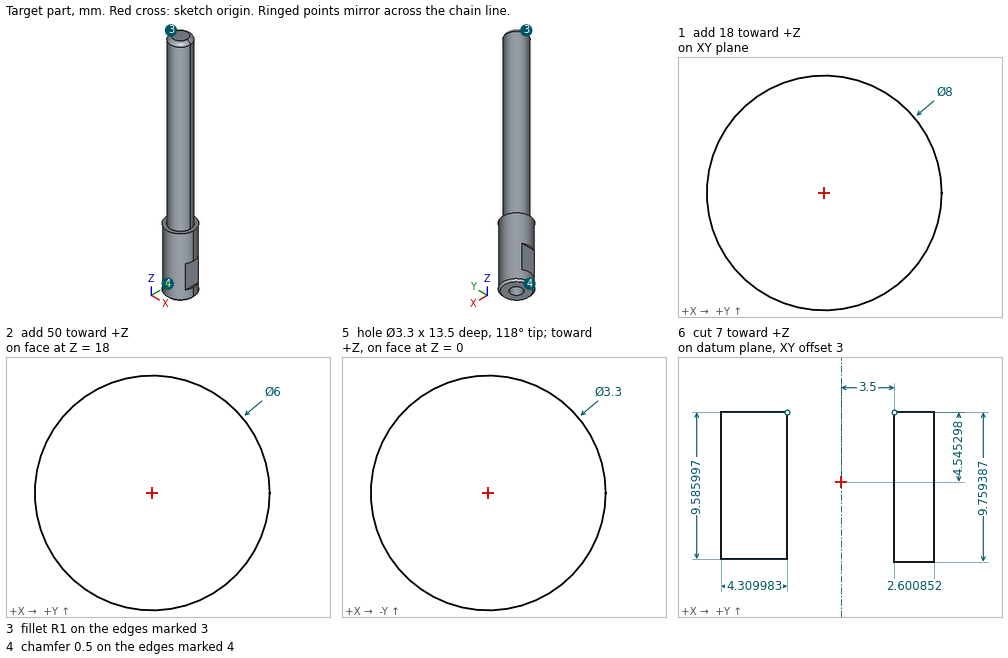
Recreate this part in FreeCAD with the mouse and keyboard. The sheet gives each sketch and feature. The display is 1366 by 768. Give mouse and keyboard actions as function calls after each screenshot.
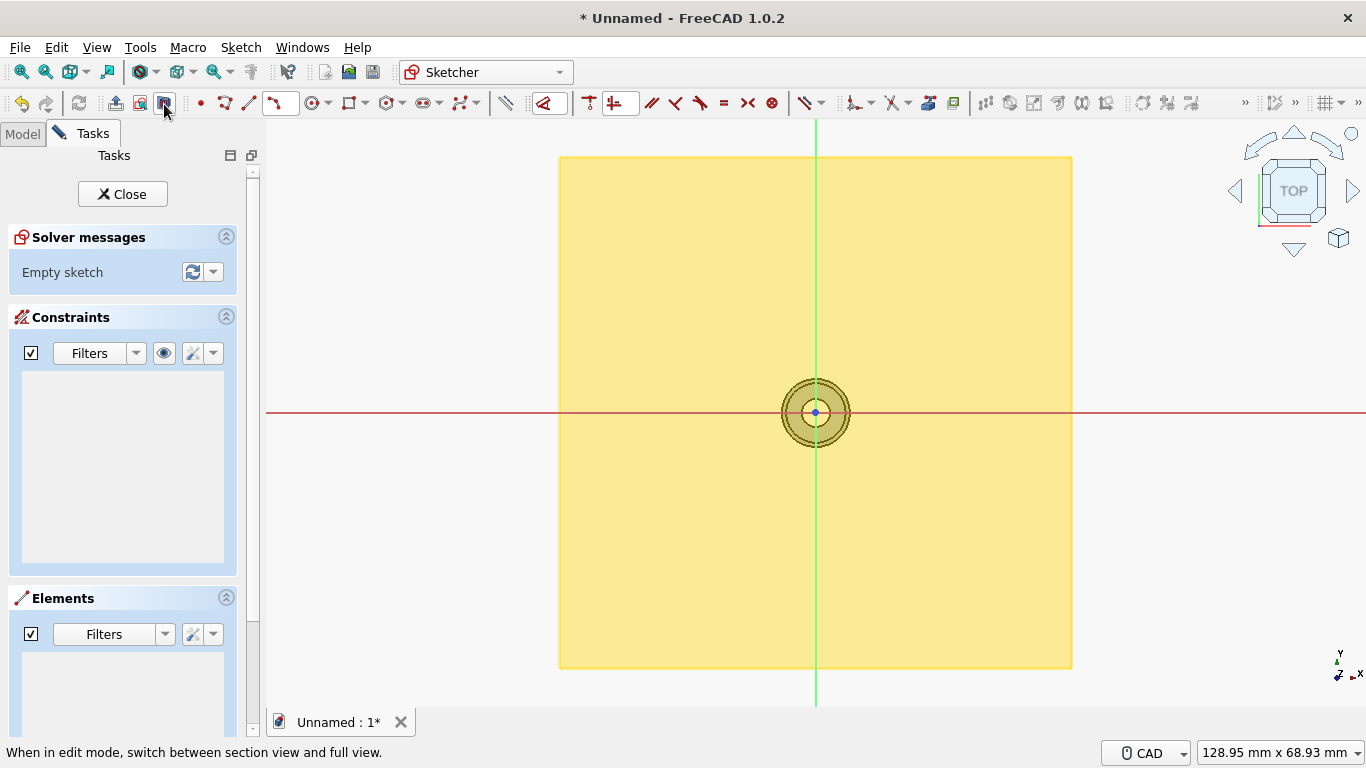
scroll(824, 417, up, 8)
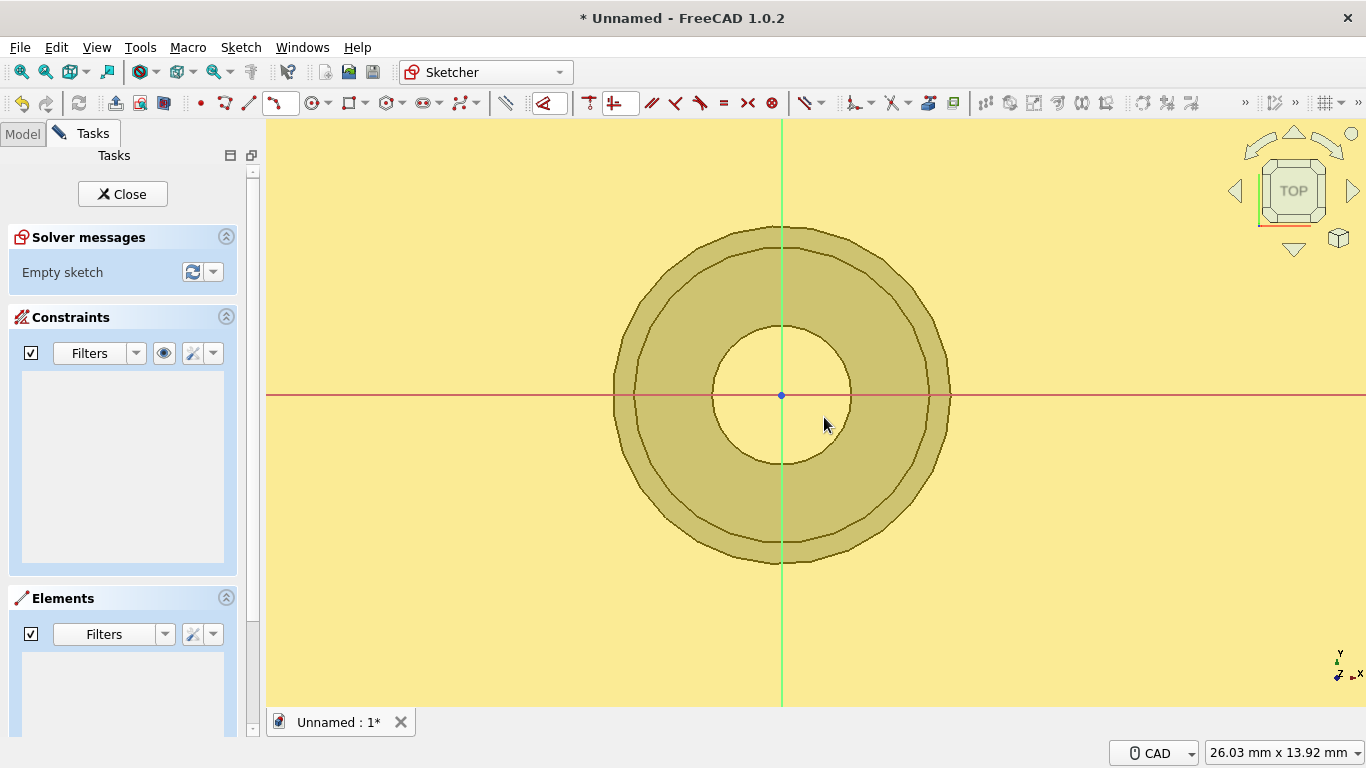
click(350, 104)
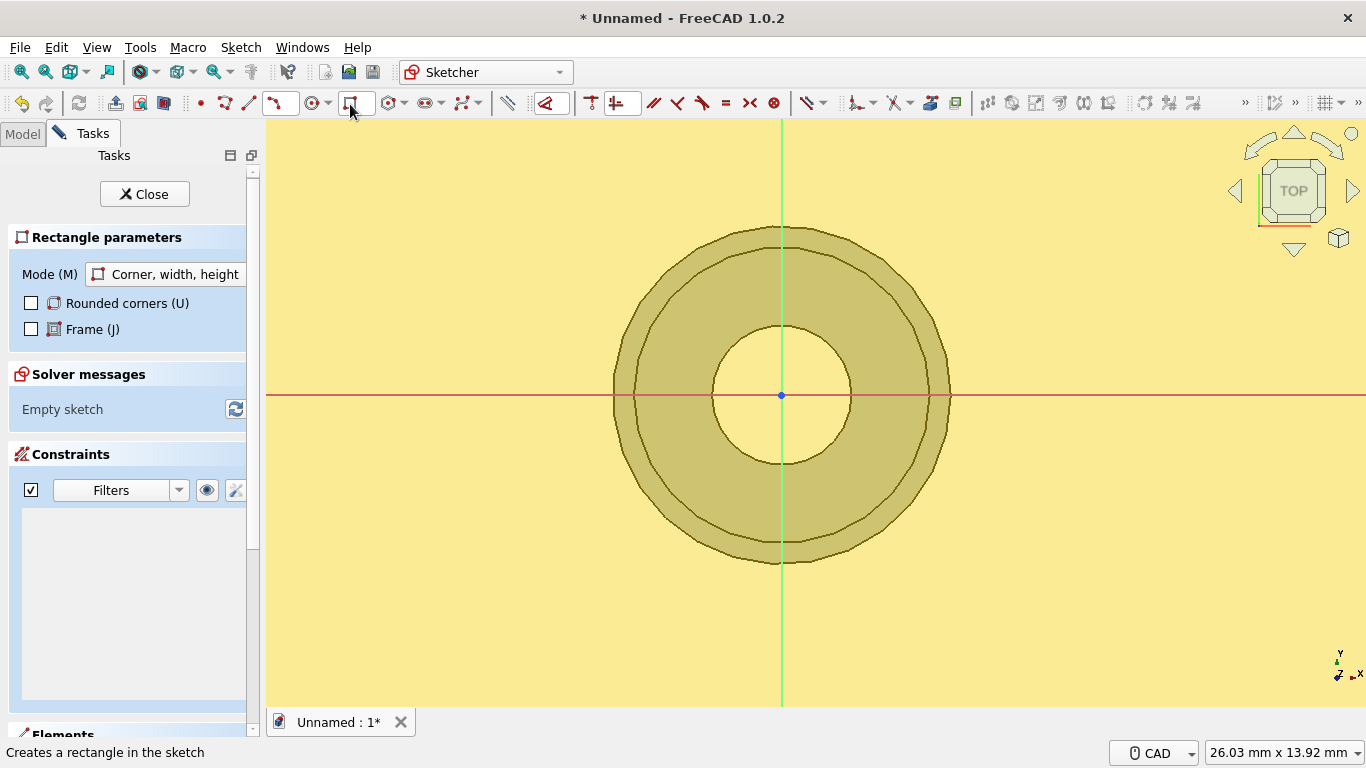
click(930, 203)
move(1040, 615)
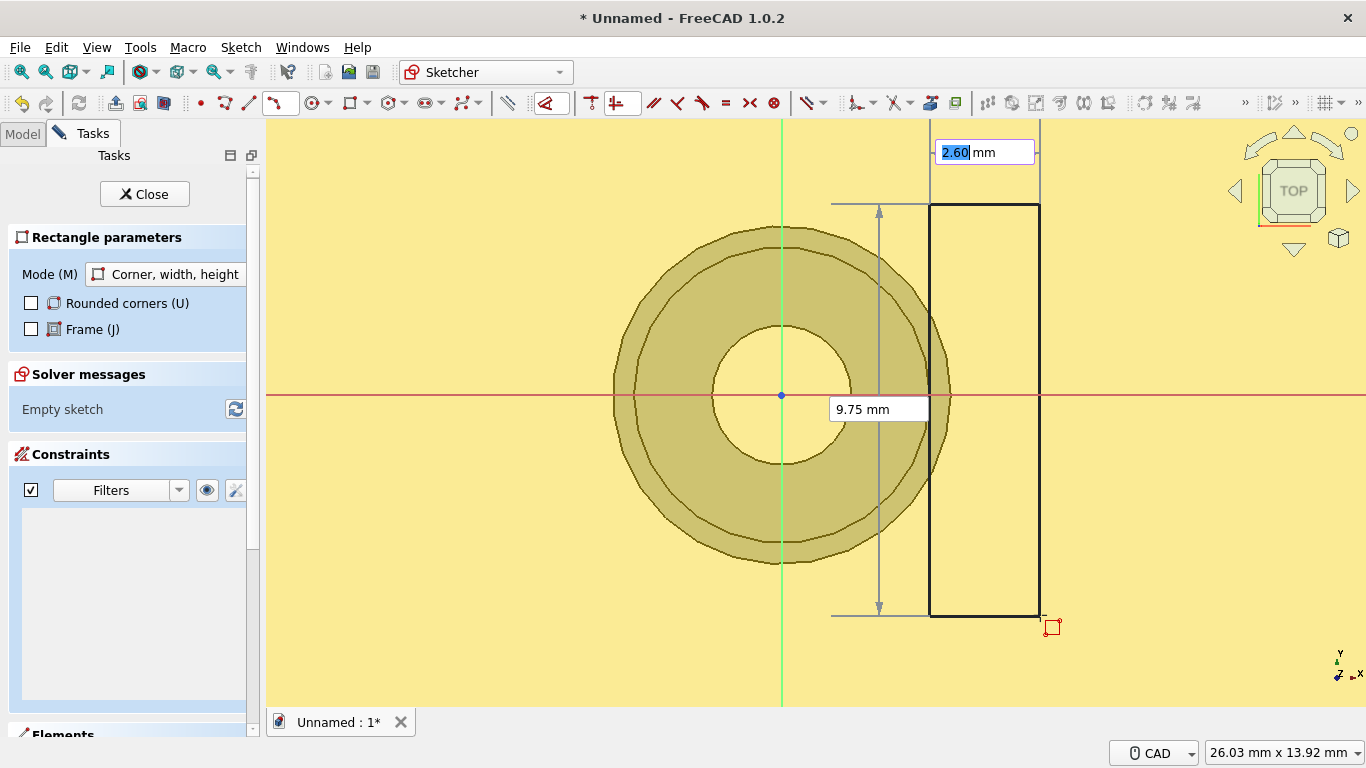
text(2.600852)
key(Tab)
text(9.759387)
key(Return)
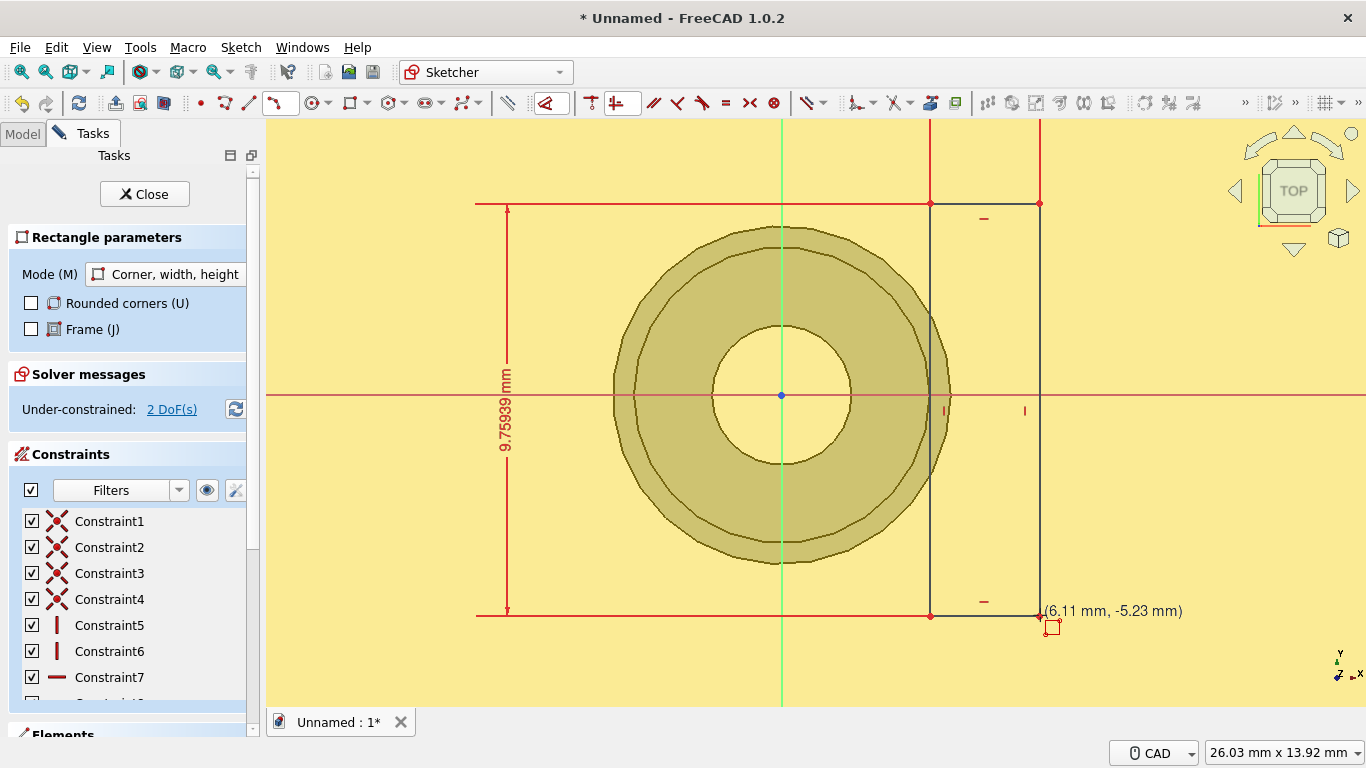
click(452, 203)
move(634, 608)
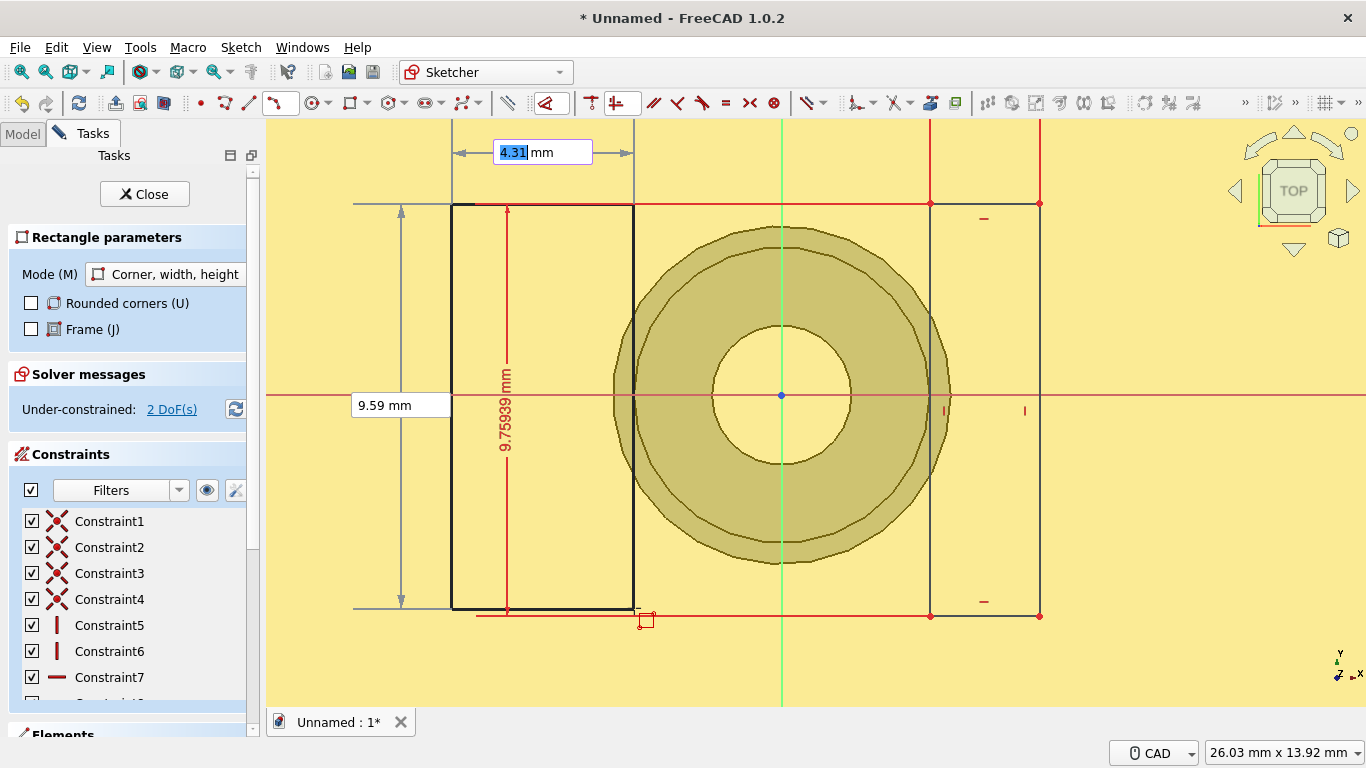
text(4.309983)
key(Tab)
text(9.585997)
key(Return)
key(Escape)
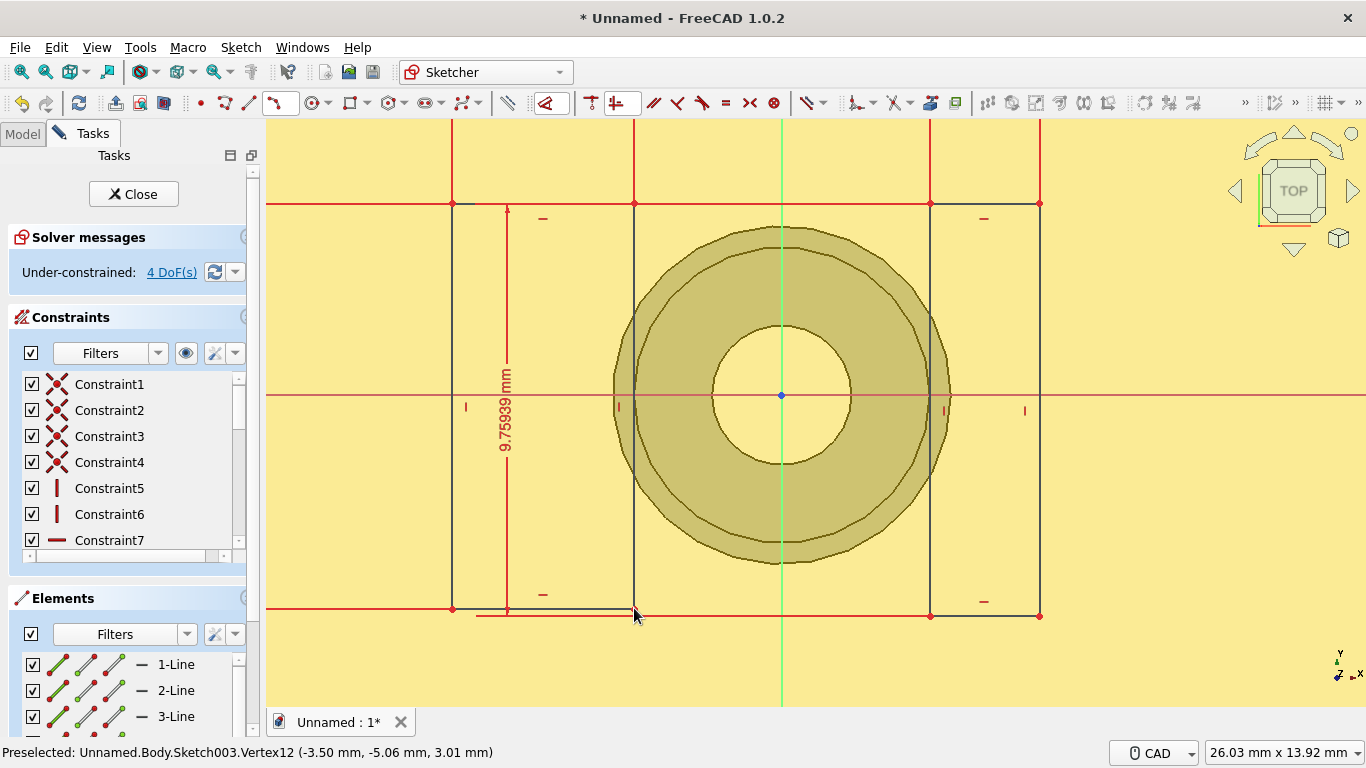
click(930, 204)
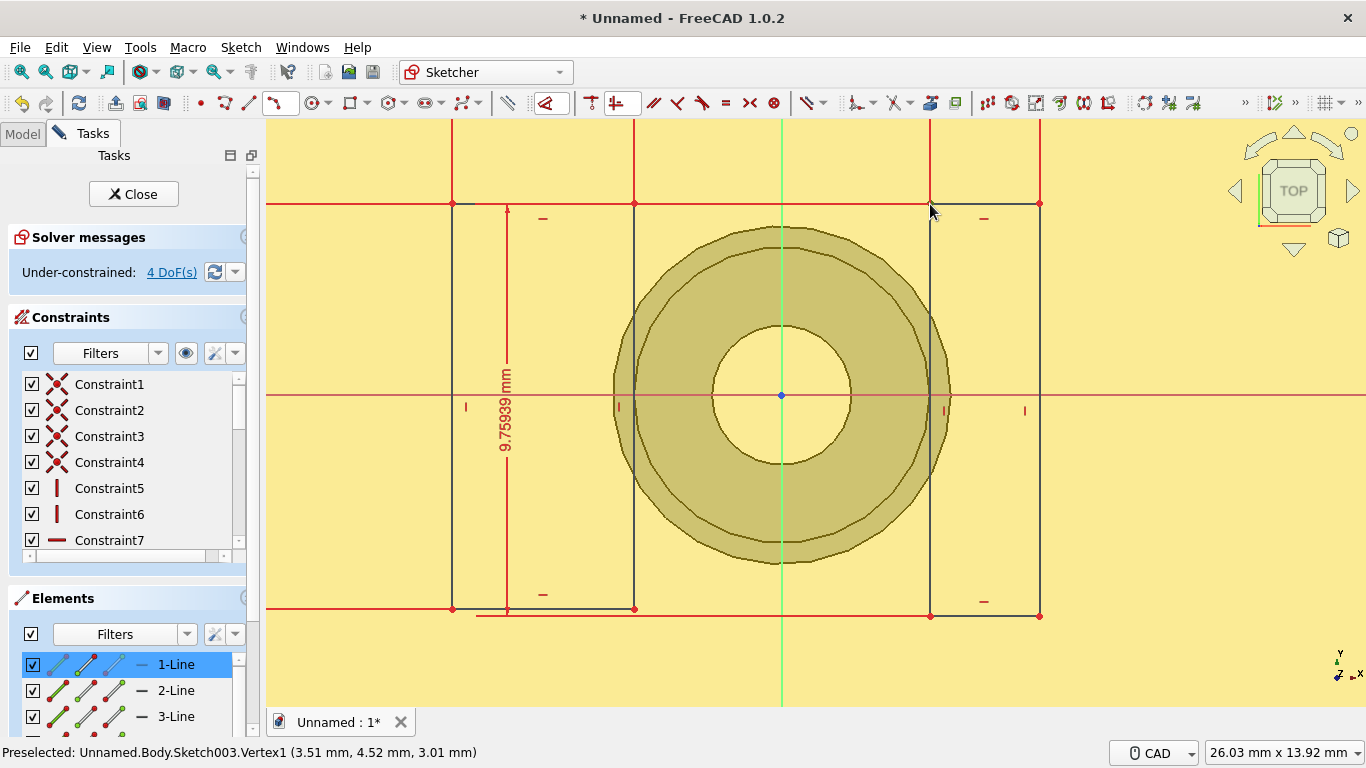
click(634, 204)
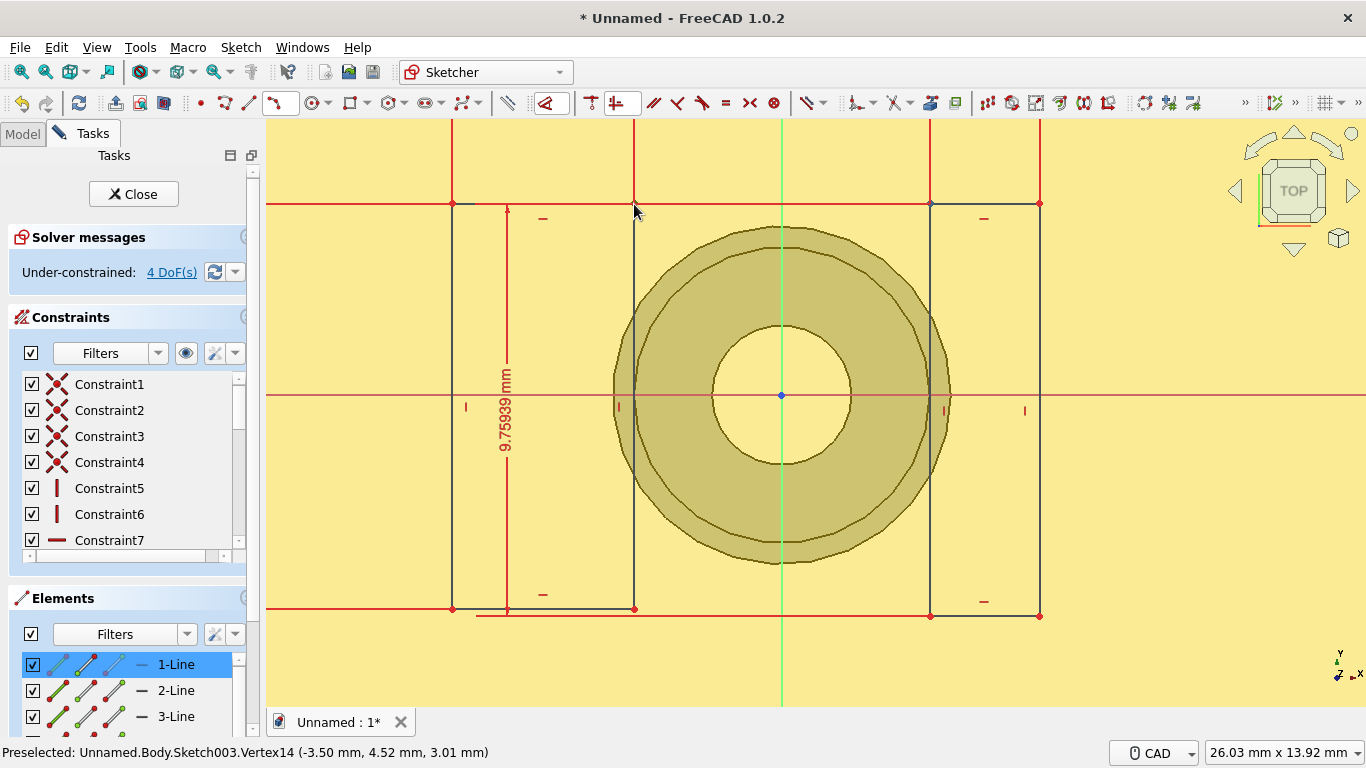
click(782, 641)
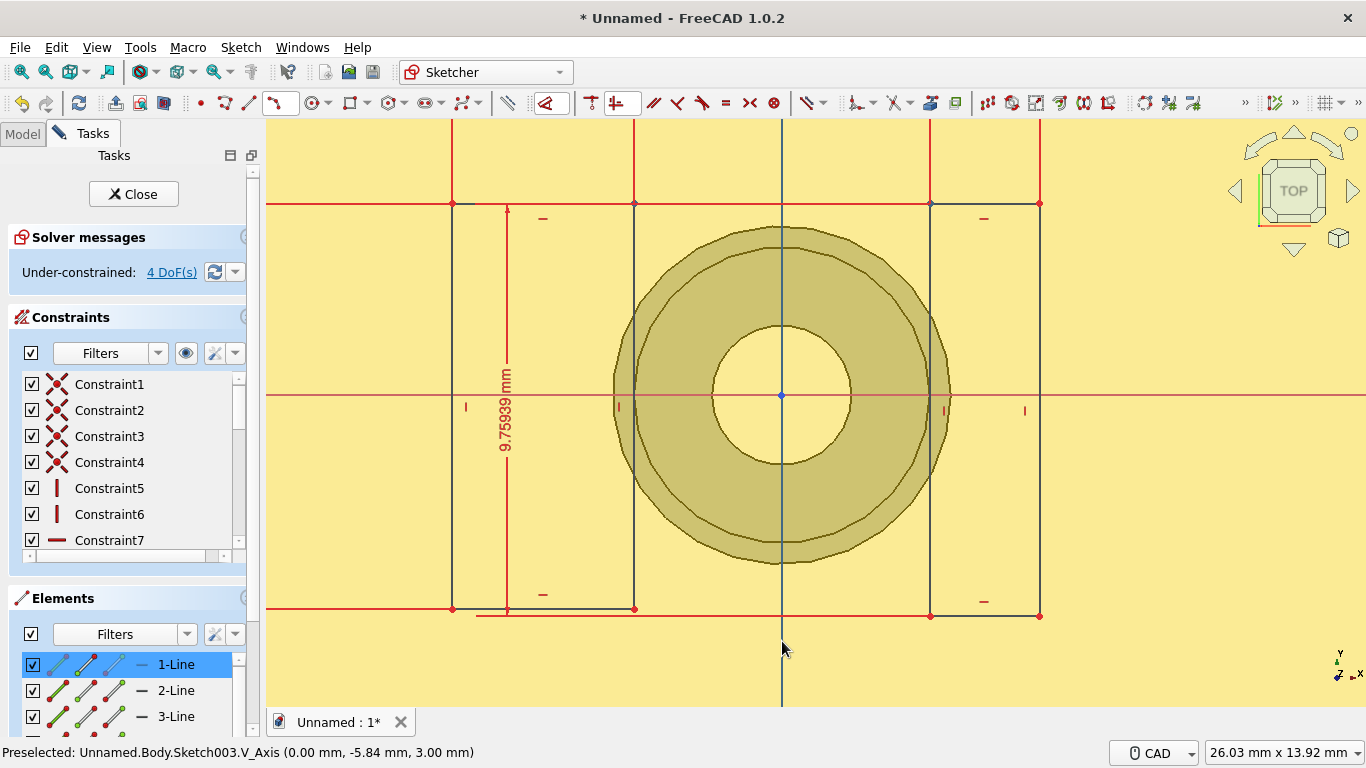
click(750, 104)